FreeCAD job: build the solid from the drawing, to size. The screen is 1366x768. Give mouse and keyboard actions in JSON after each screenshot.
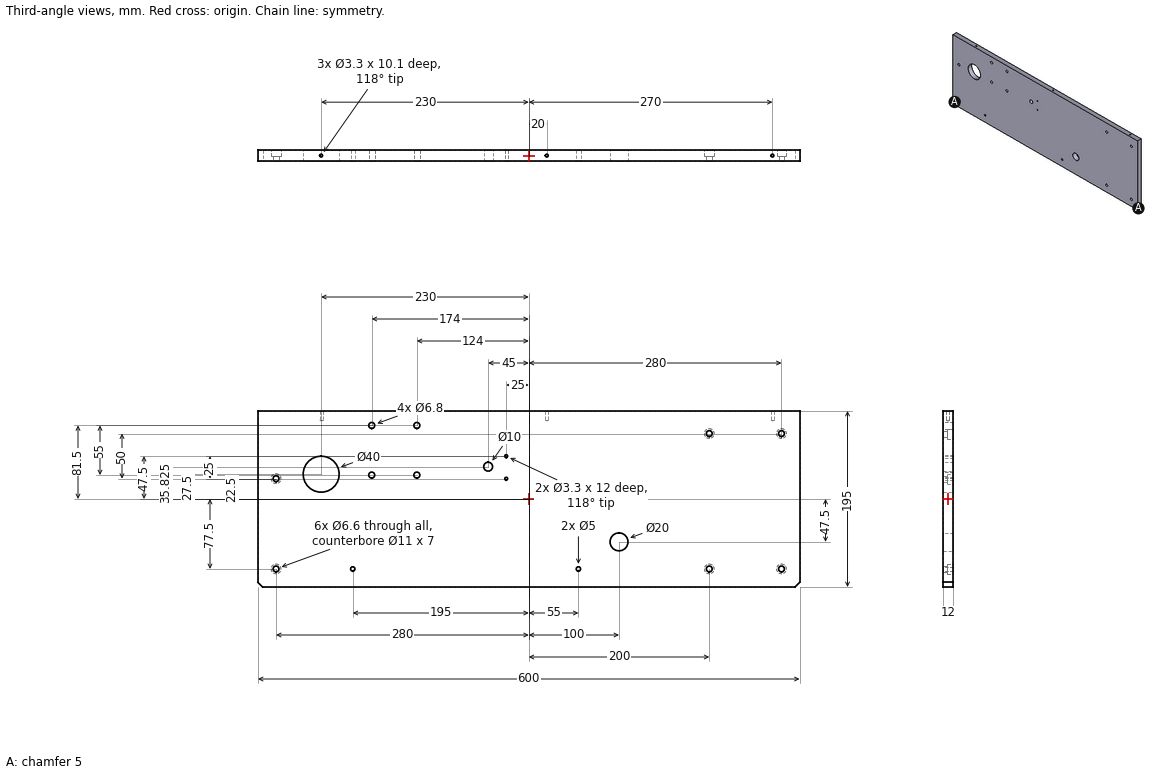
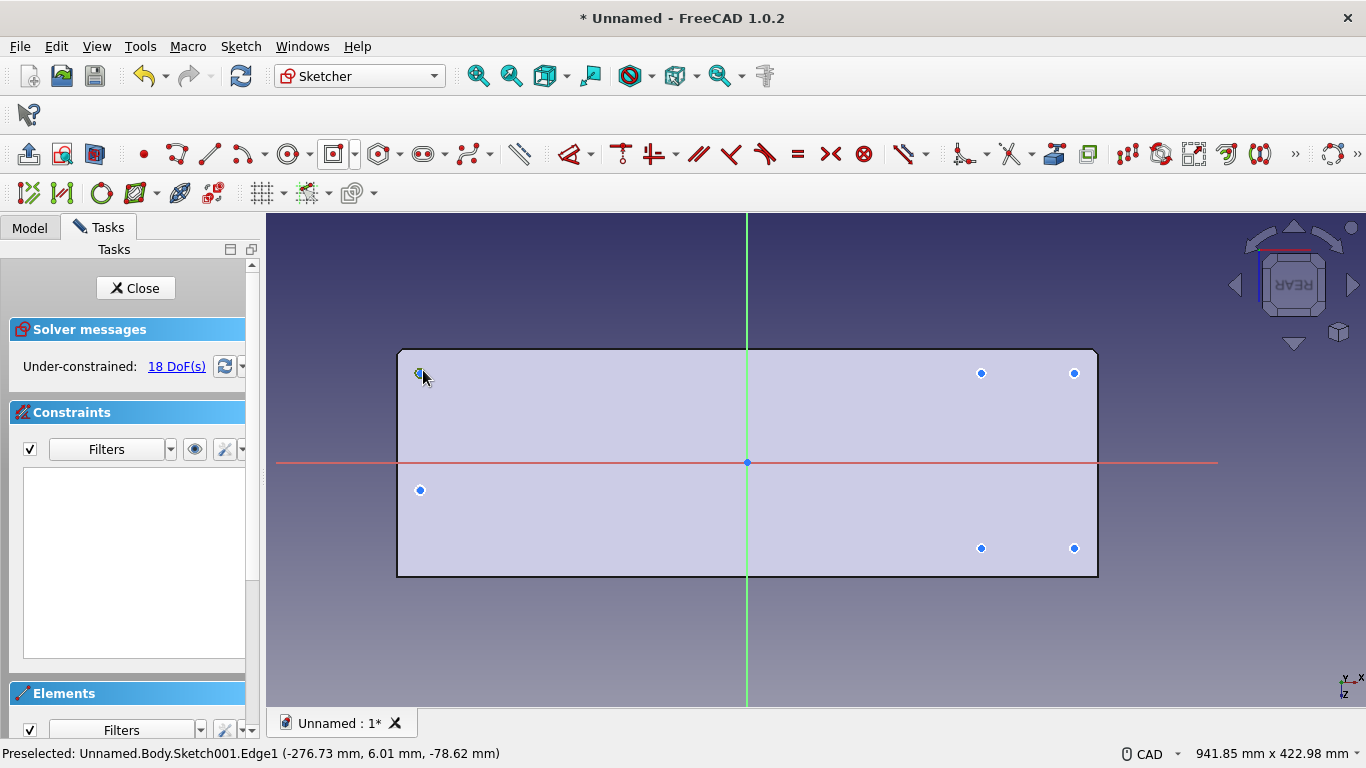
{"action": "scroll", "coordinate": [424, 487], "scroll_direction": "up", "scroll_amount": 6}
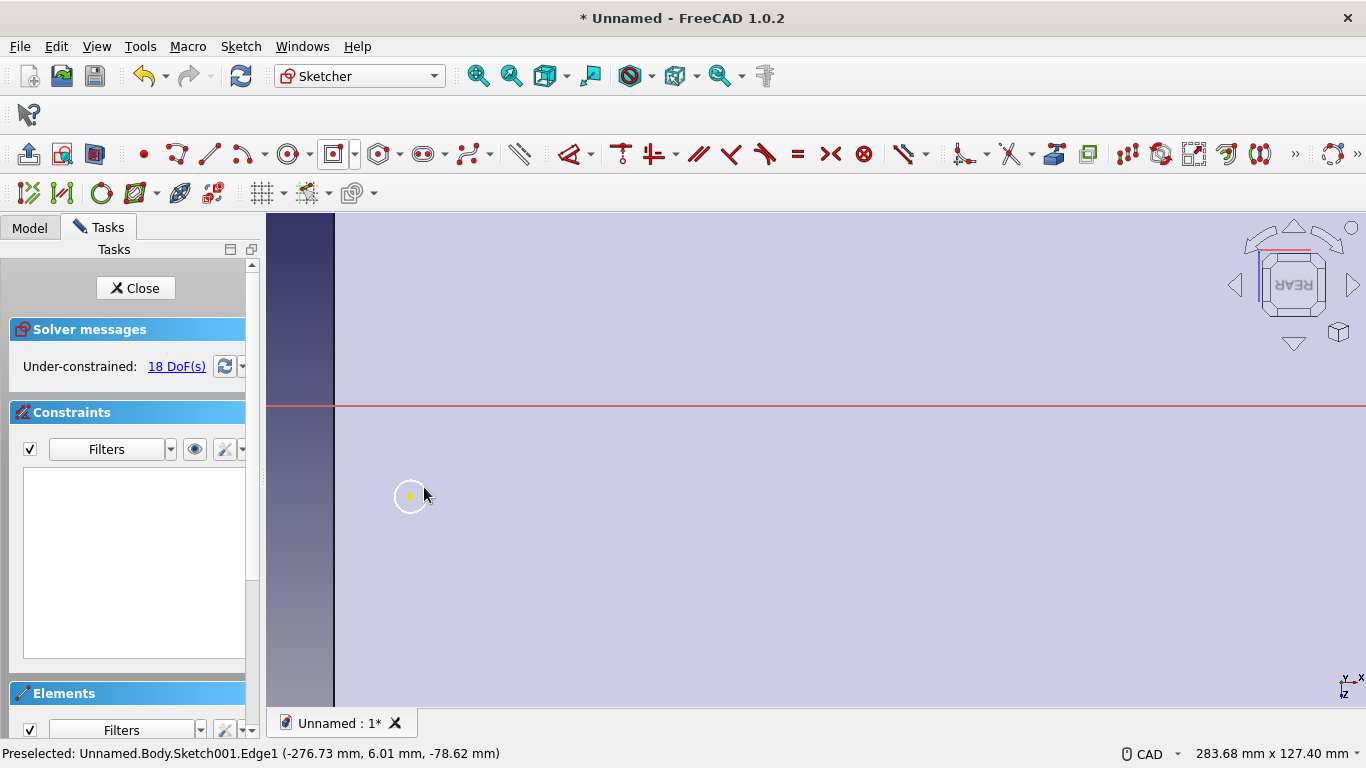
{"action": "left_click", "coordinate": [422, 485]}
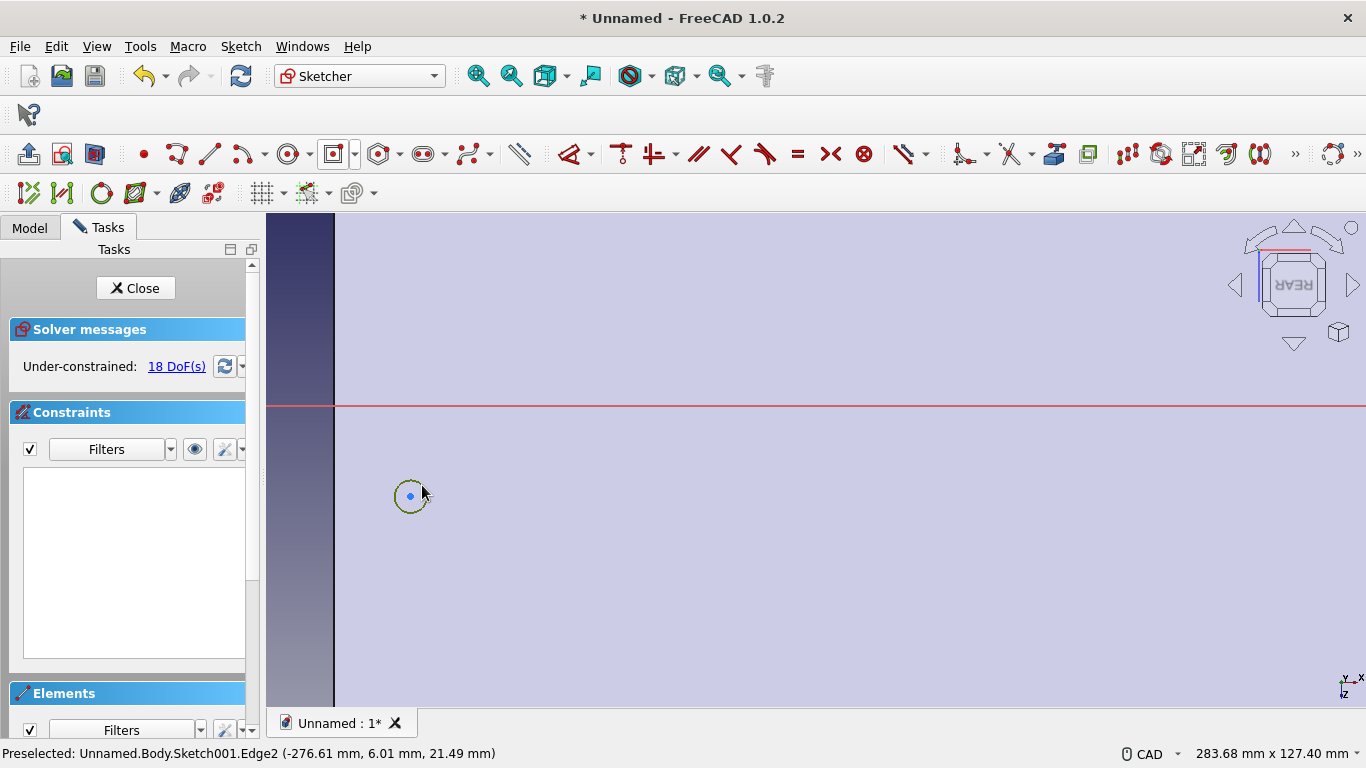
{"action": "scroll", "coordinate": [424, 488], "scroll_direction": "down", "scroll_amount": 6}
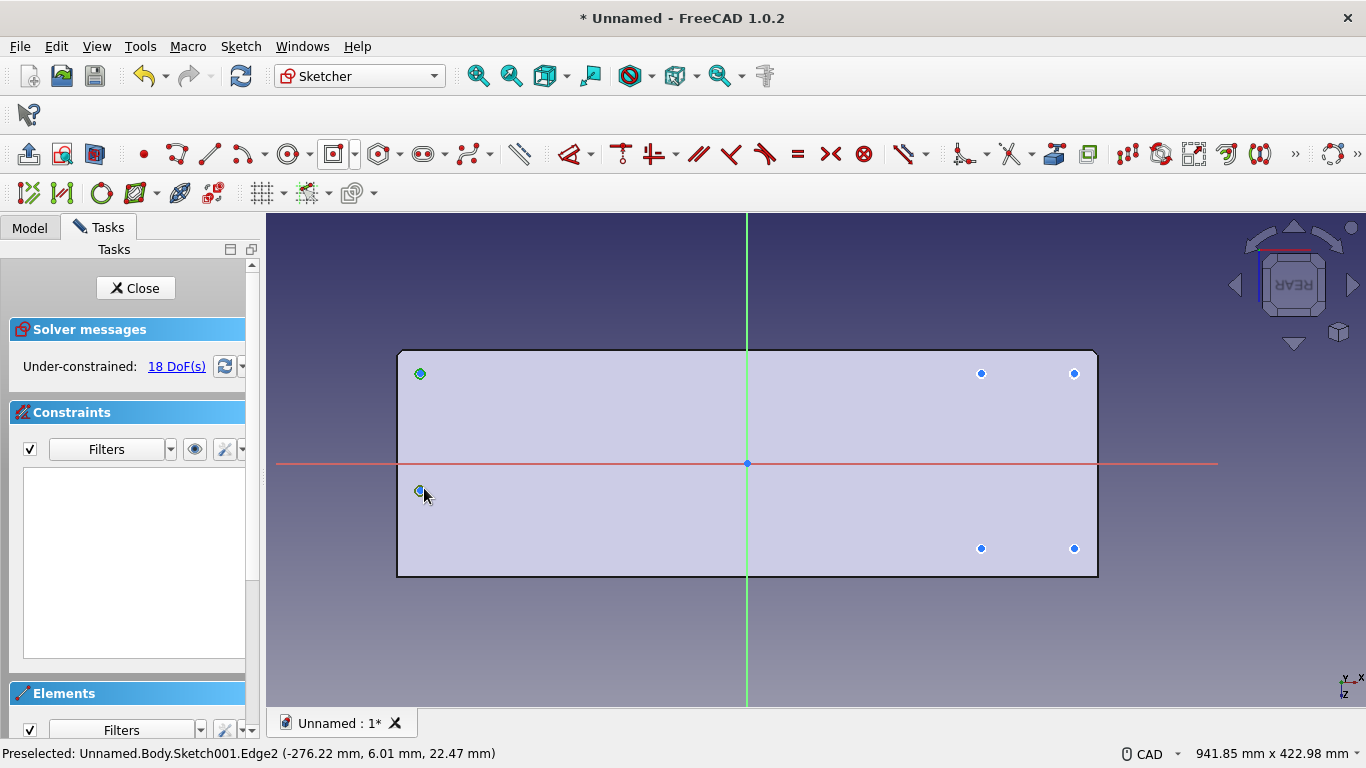
{"action": "scroll", "coordinate": [984, 371], "scroll_direction": "up", "scroll_amount": 6}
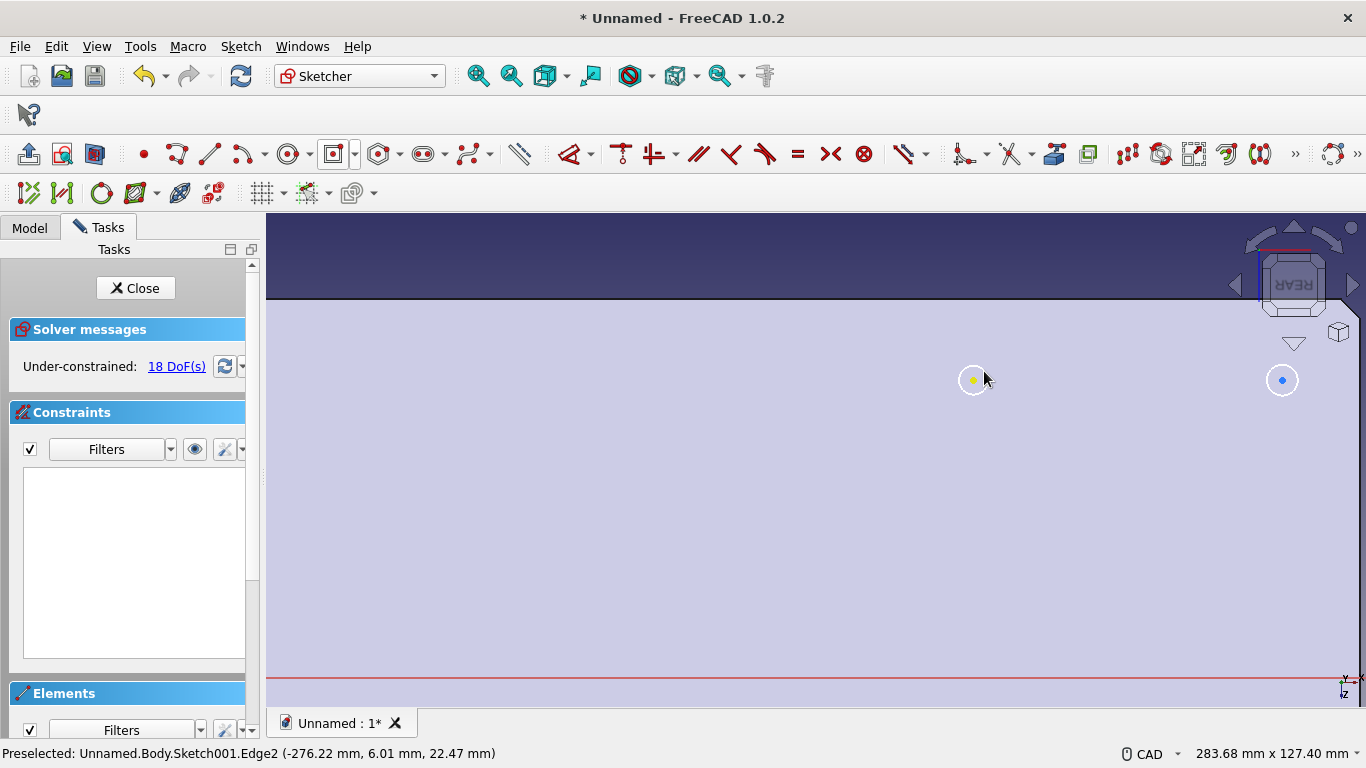
{"action": "left_click", "coordinate": [984, 370]}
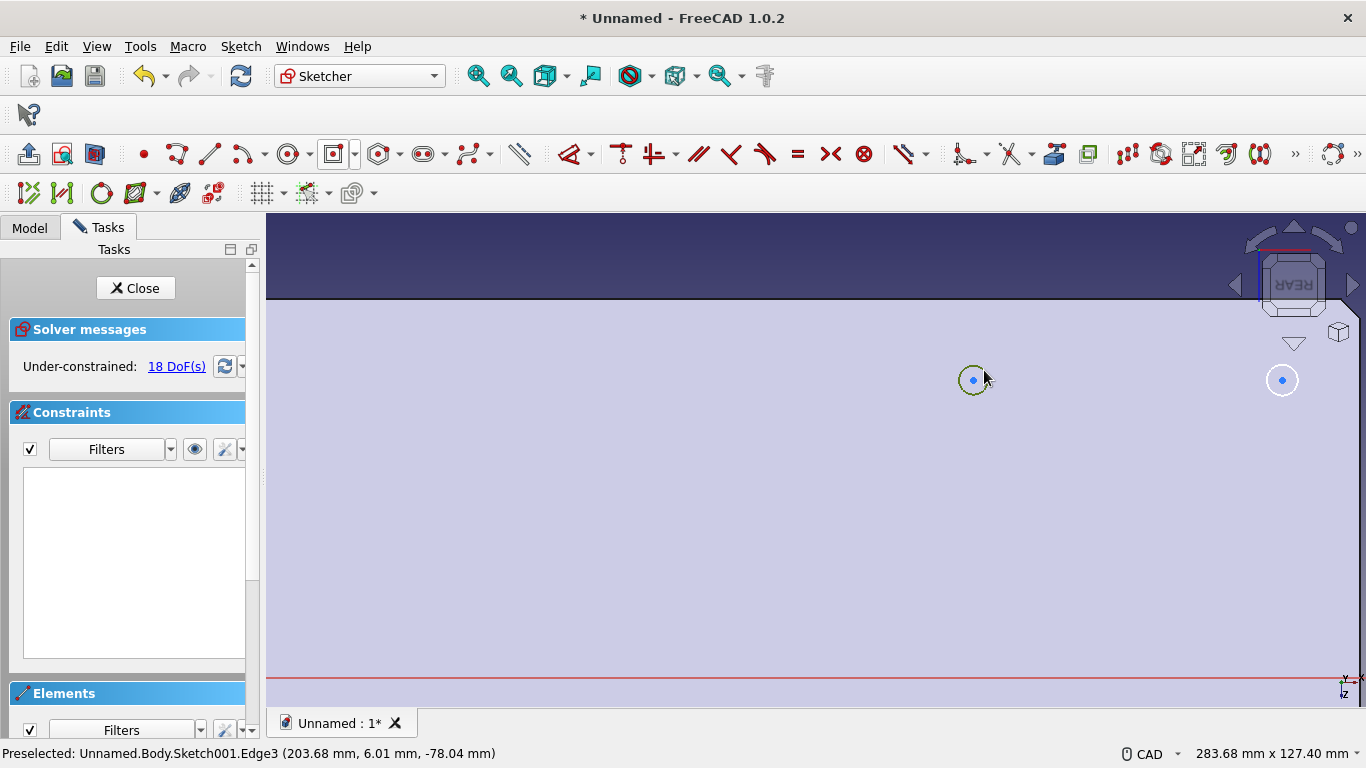
{"action": "scroll", "coordinate": [985, 370], "scroll_direction": "down", "scroll_amount": 6}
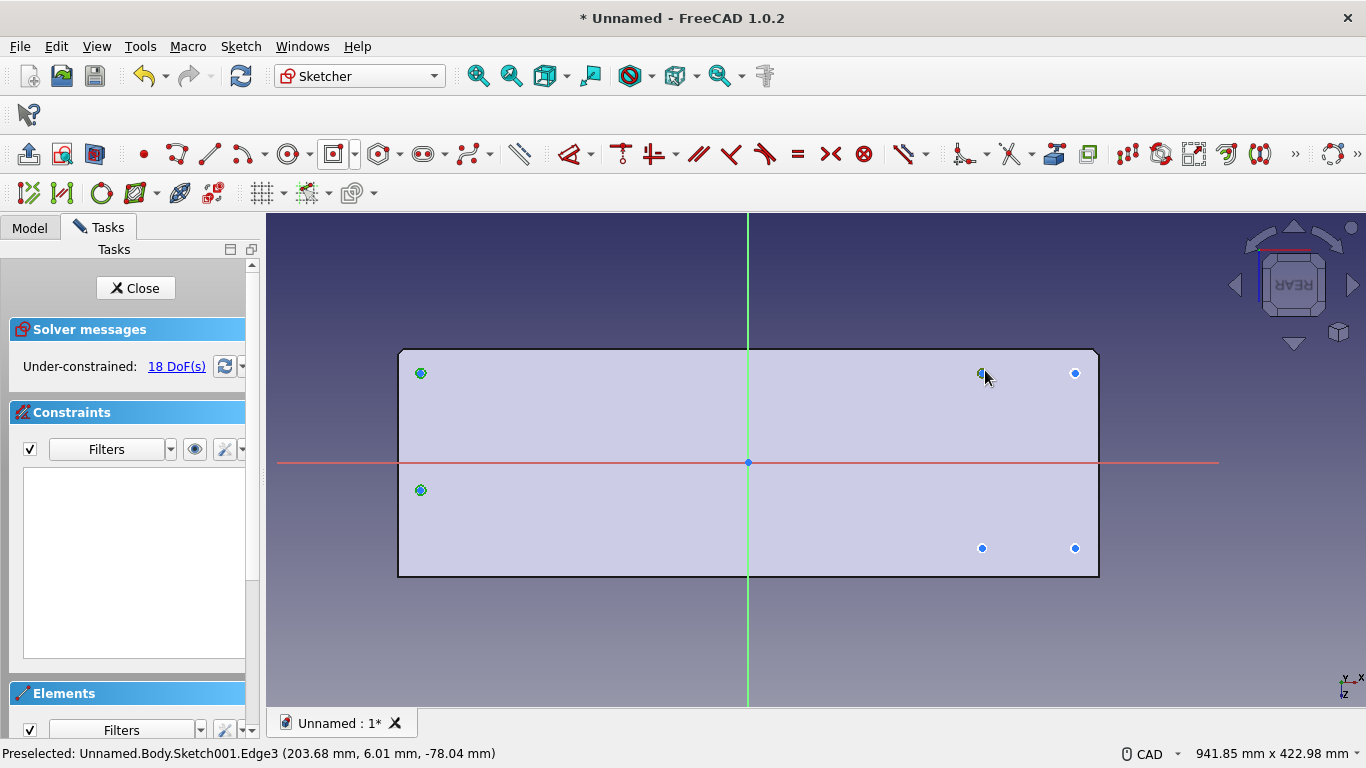
{"action": "scroll", "coordinate": [1078, 370], "scroll_direction": "up", "scroll_amount": 6}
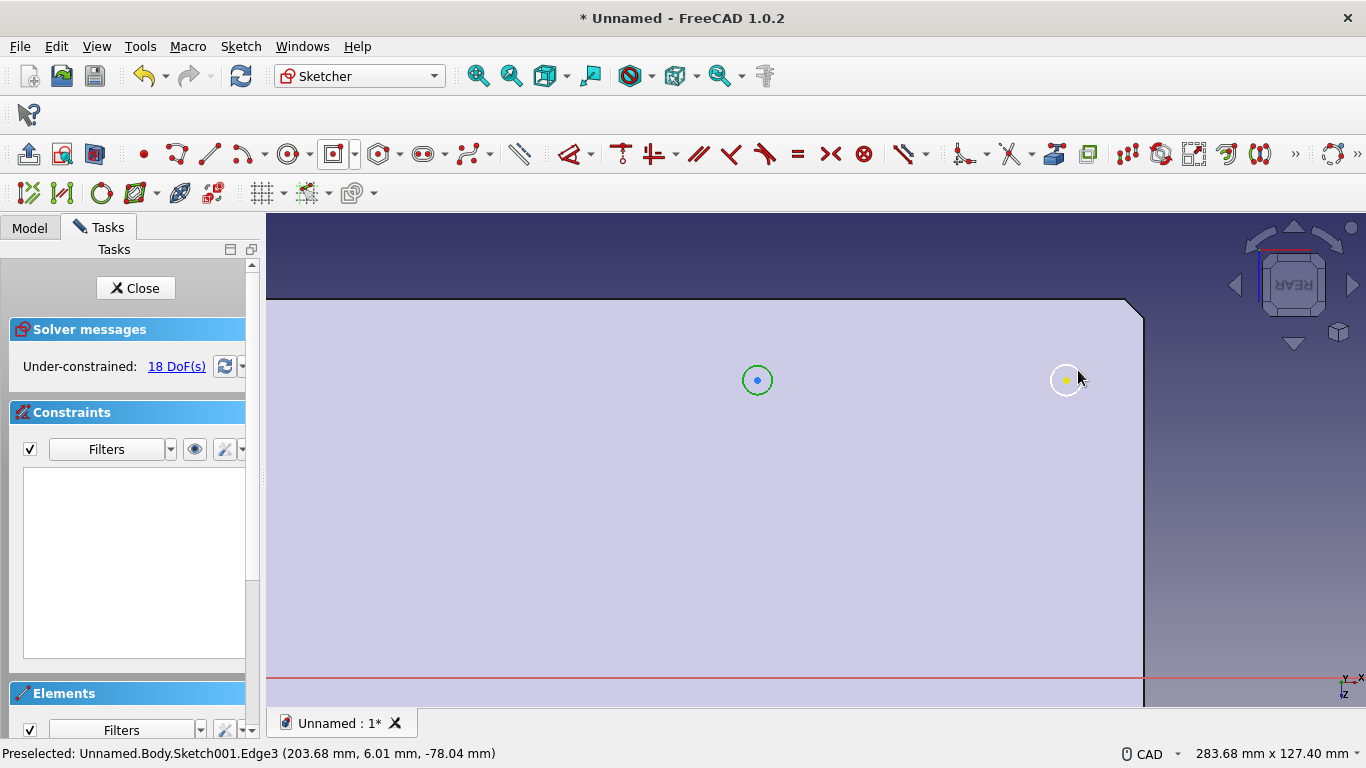
{"action": "left_click", "coordinate": [1077, 369]}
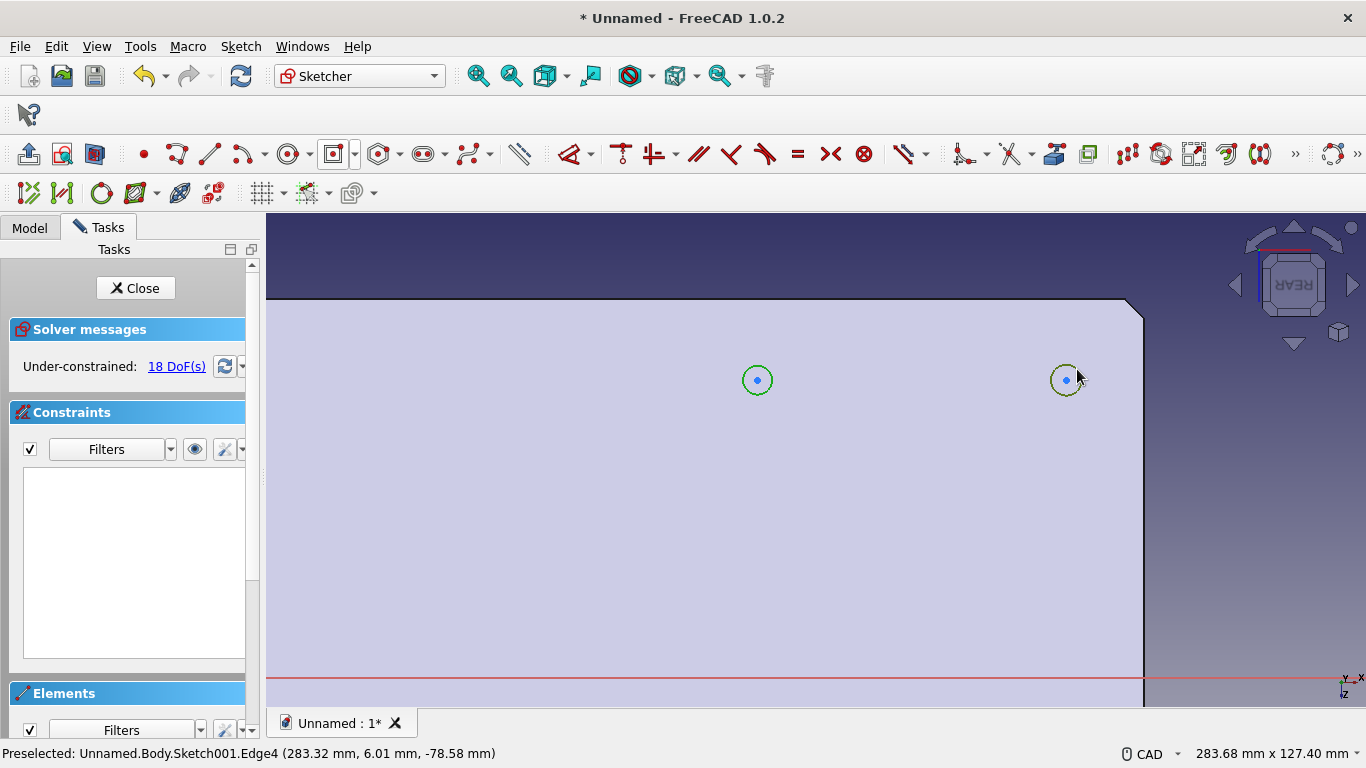
{"action": "scroll", "coordinate": [1078, 370], "scroll_direction": "down", "scroll_amount": 6}